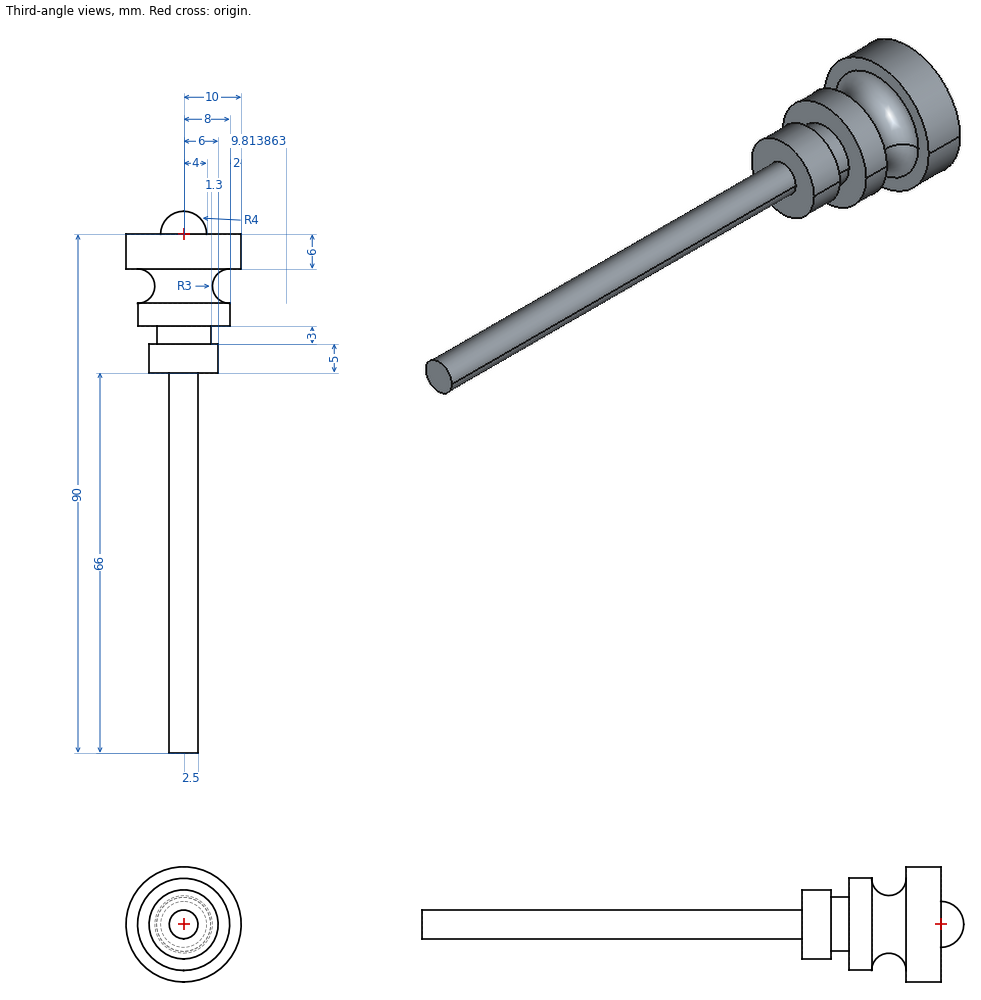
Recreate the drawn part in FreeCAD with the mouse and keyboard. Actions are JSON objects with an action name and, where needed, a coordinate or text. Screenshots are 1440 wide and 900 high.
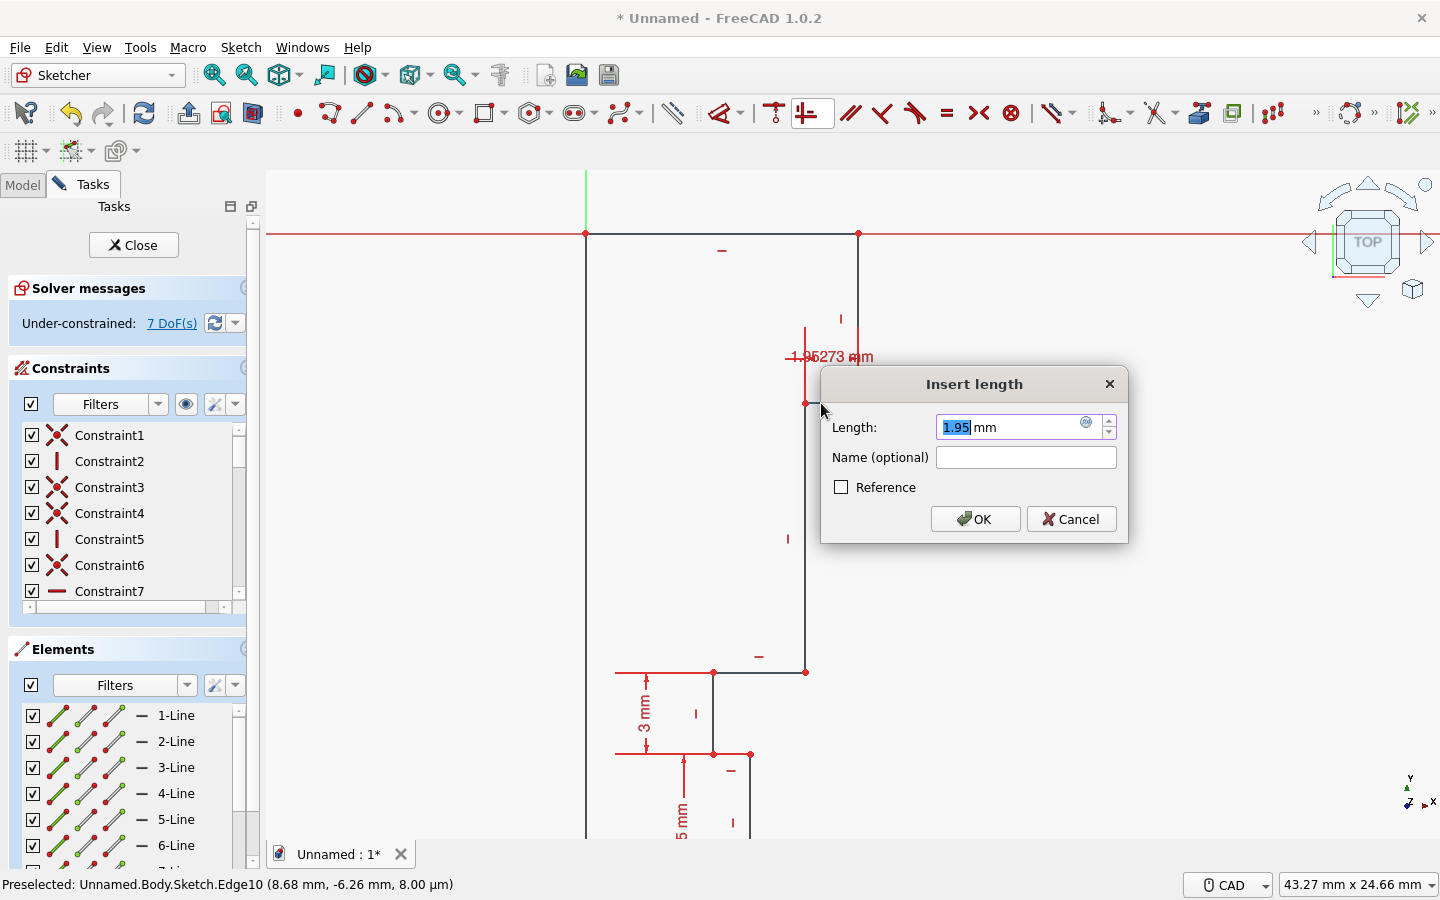
{"action": "type", "text": "2"}
{"action": "key", "text": "Return"}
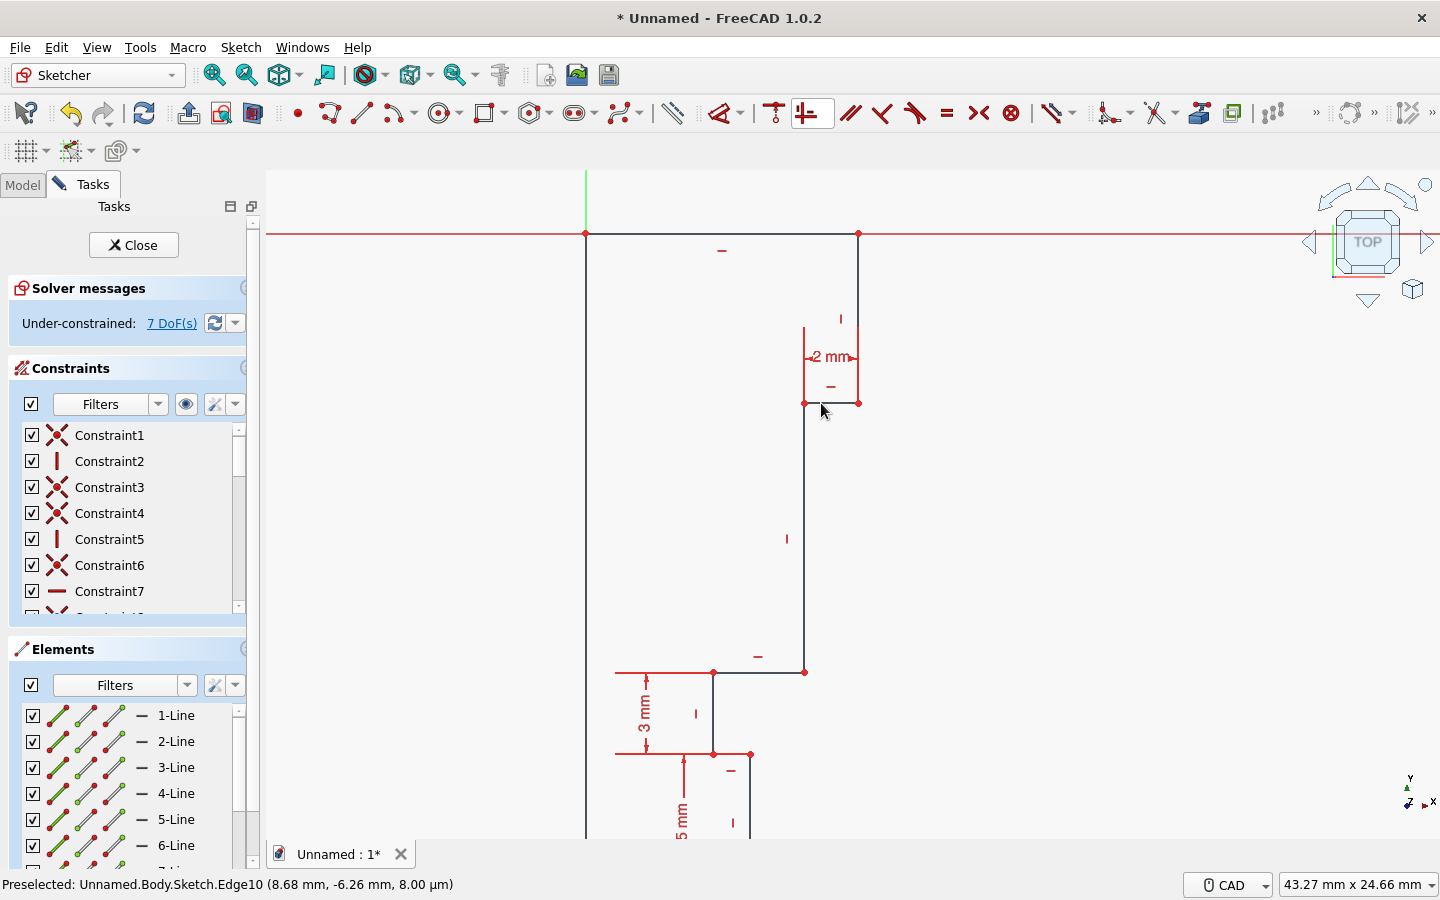
{"action": "scroll", "coordinate": [797, 316], "scroll_direction": "down", "scroll_amount": 9}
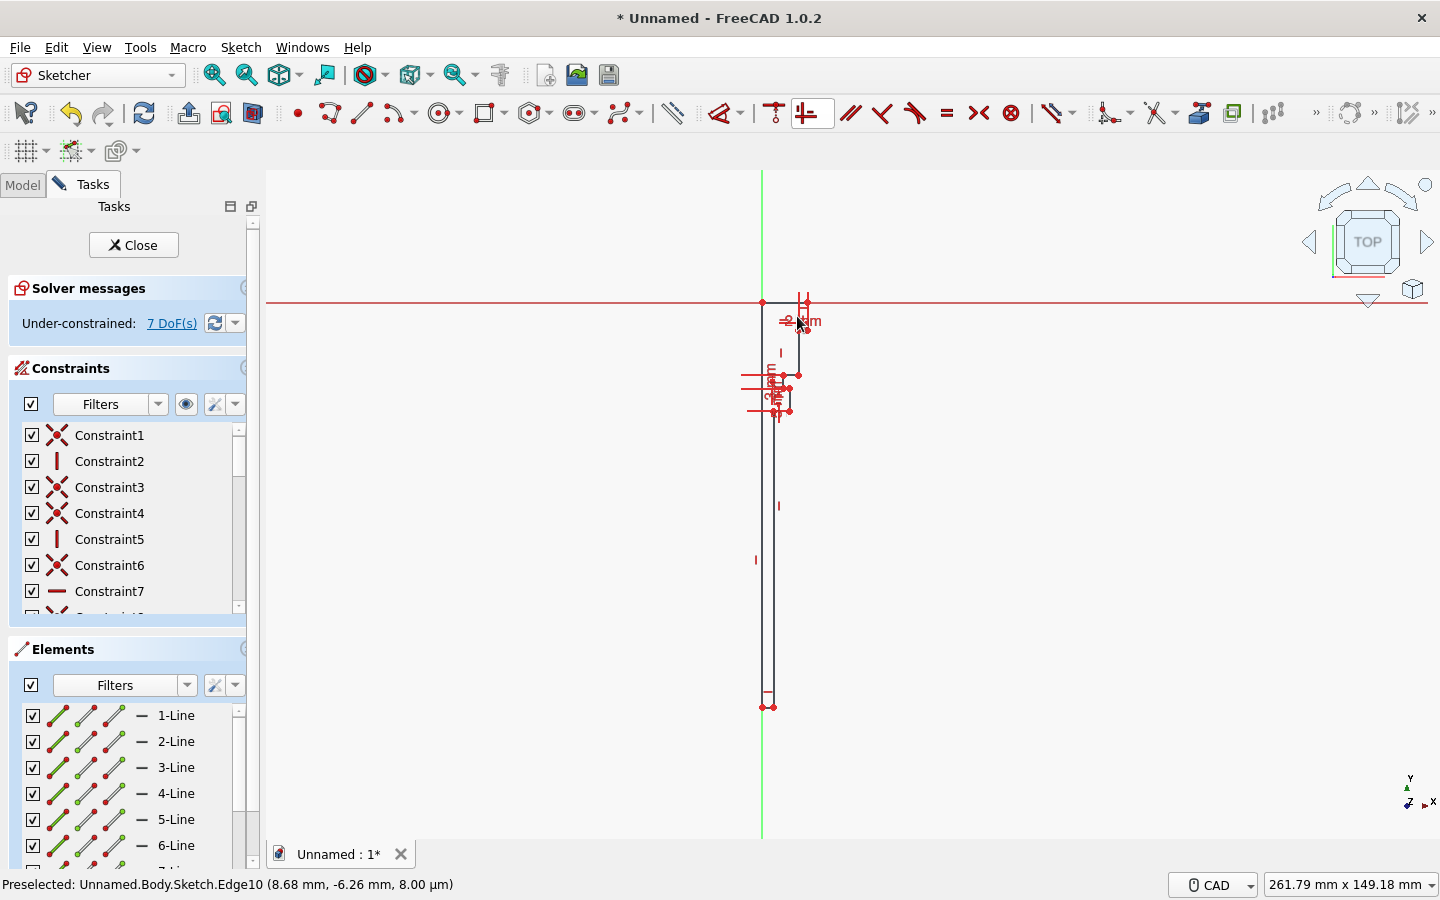
{"action": "scroll", "coordinate": [808, 322], "scroll_direction": "up", "scroll_amount": 3}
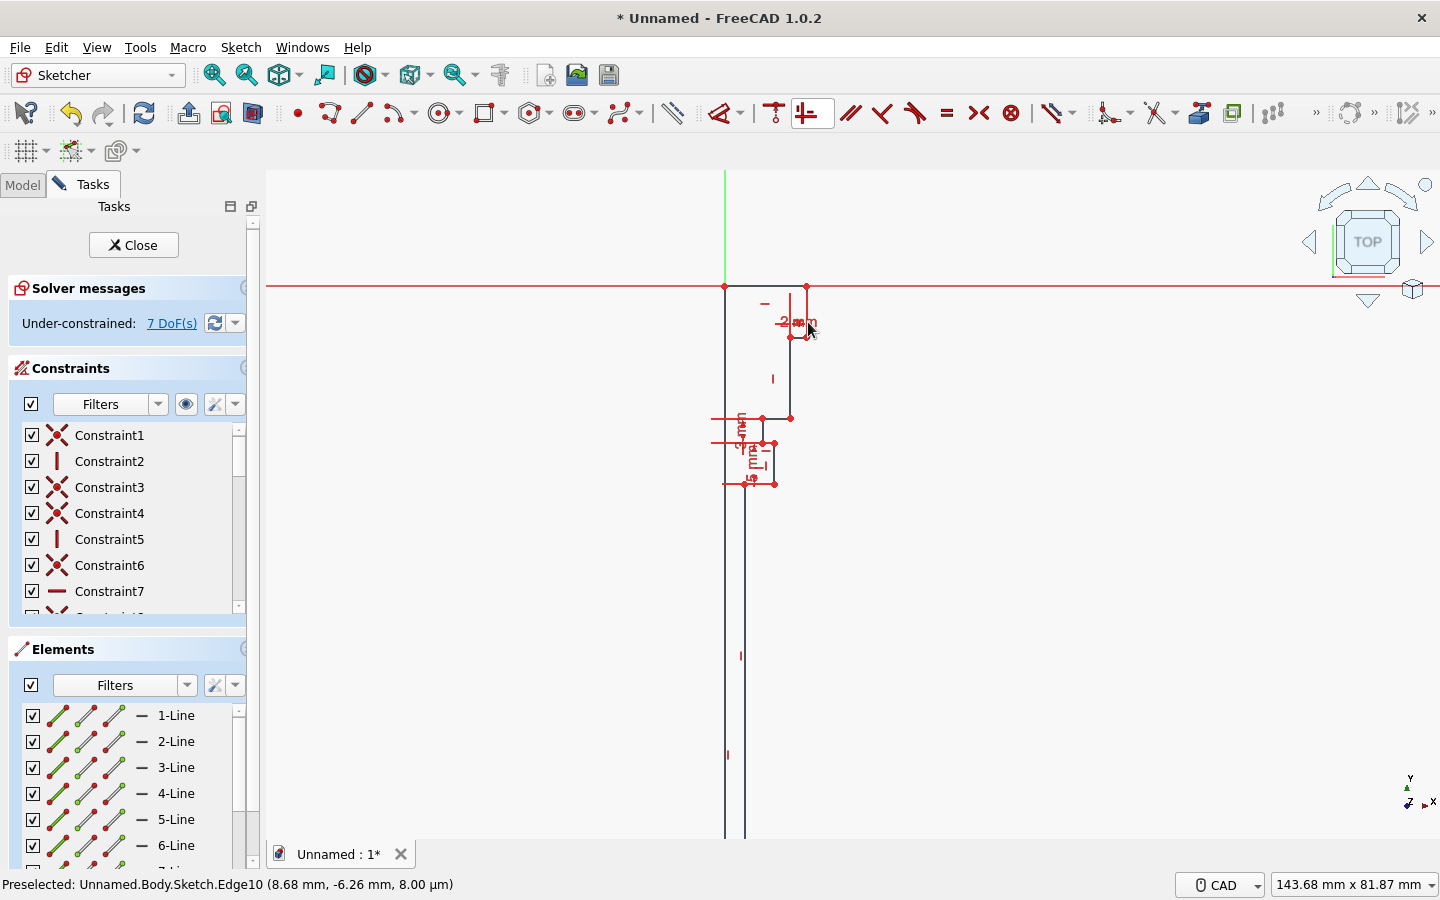
{"action": "left_click", "coordinate": [807, 302]}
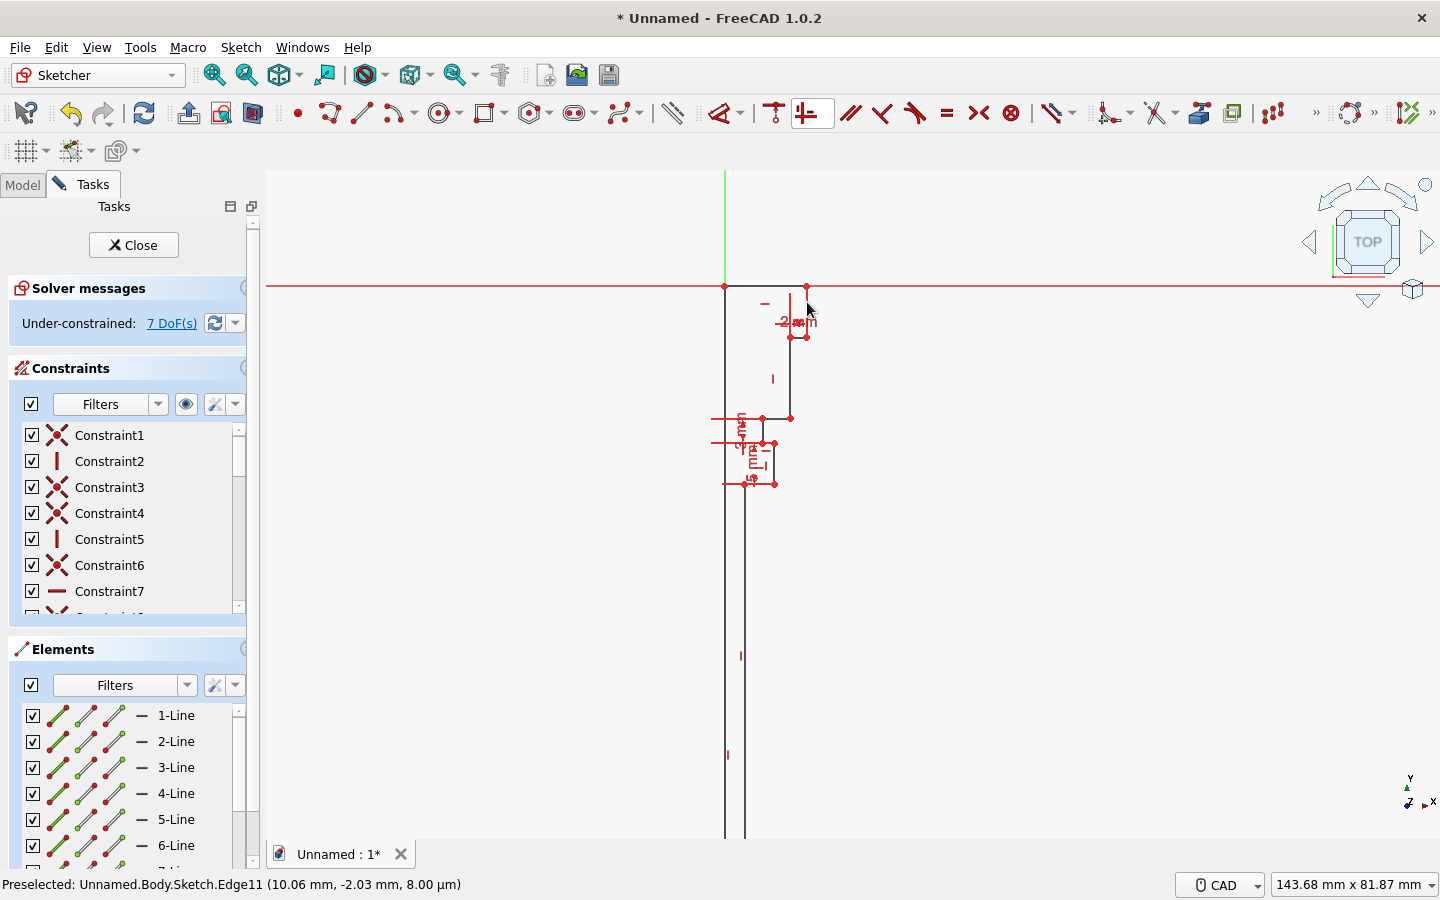
{"action": "key", "text": "i"}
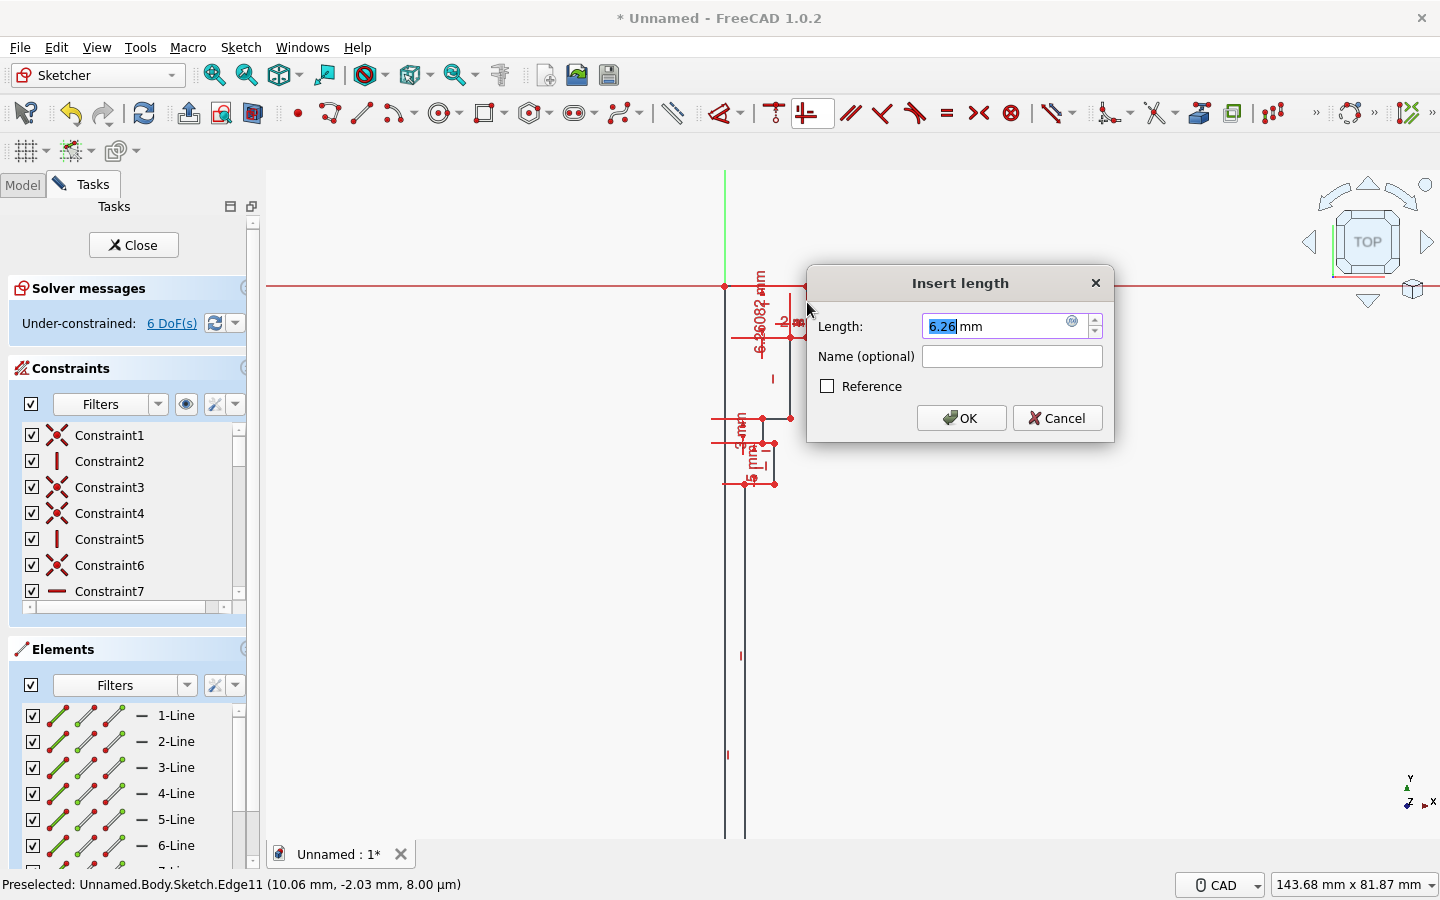
{"action": "type", "text": "6"}
{"action": "key", "text": "Return"}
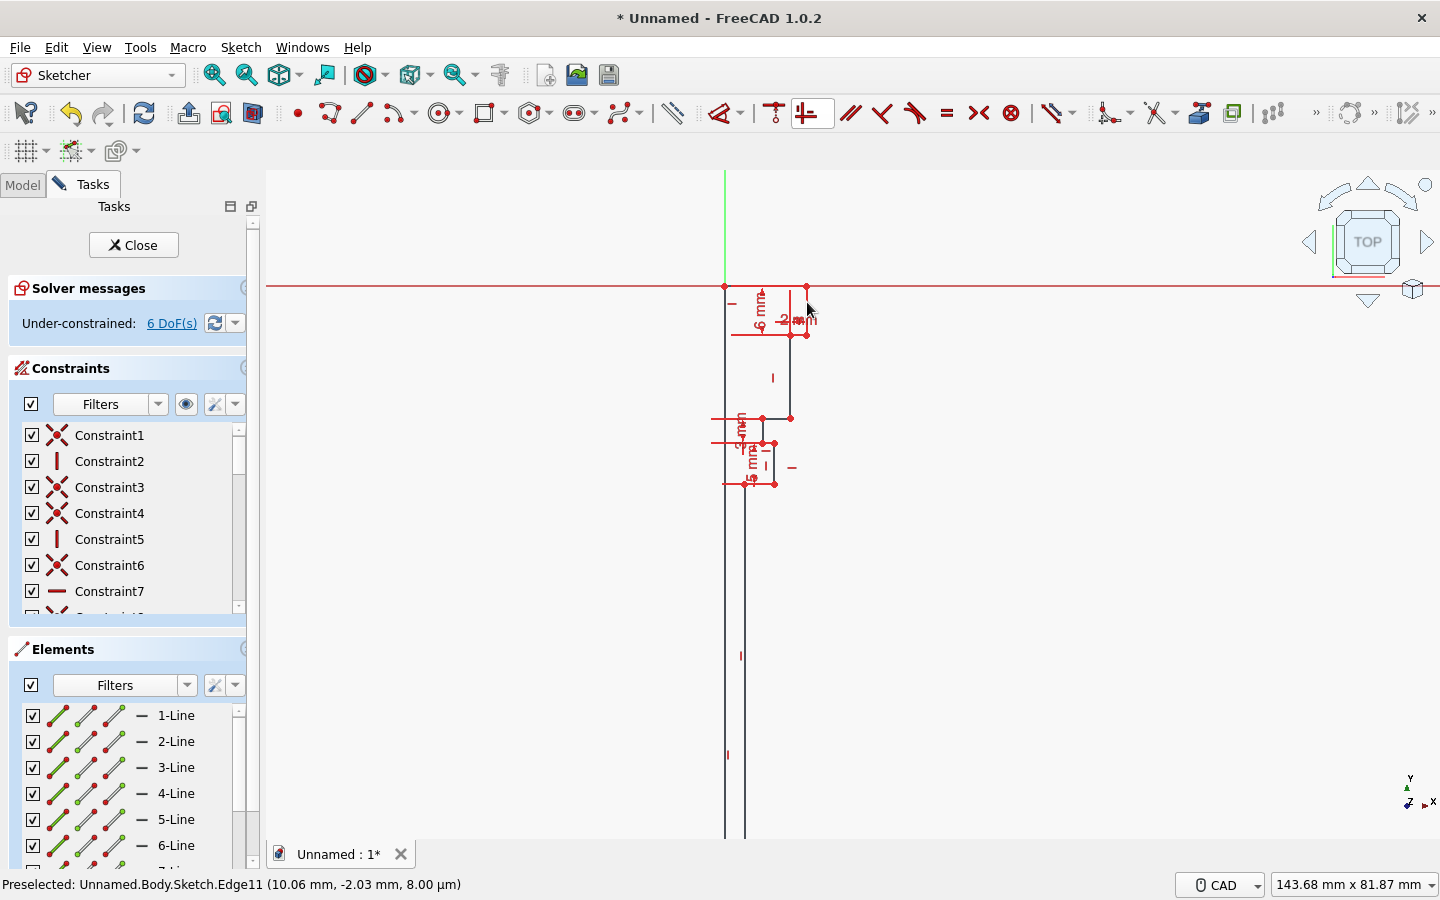
{"action": "left_click", "coordinate": [725, 508]}